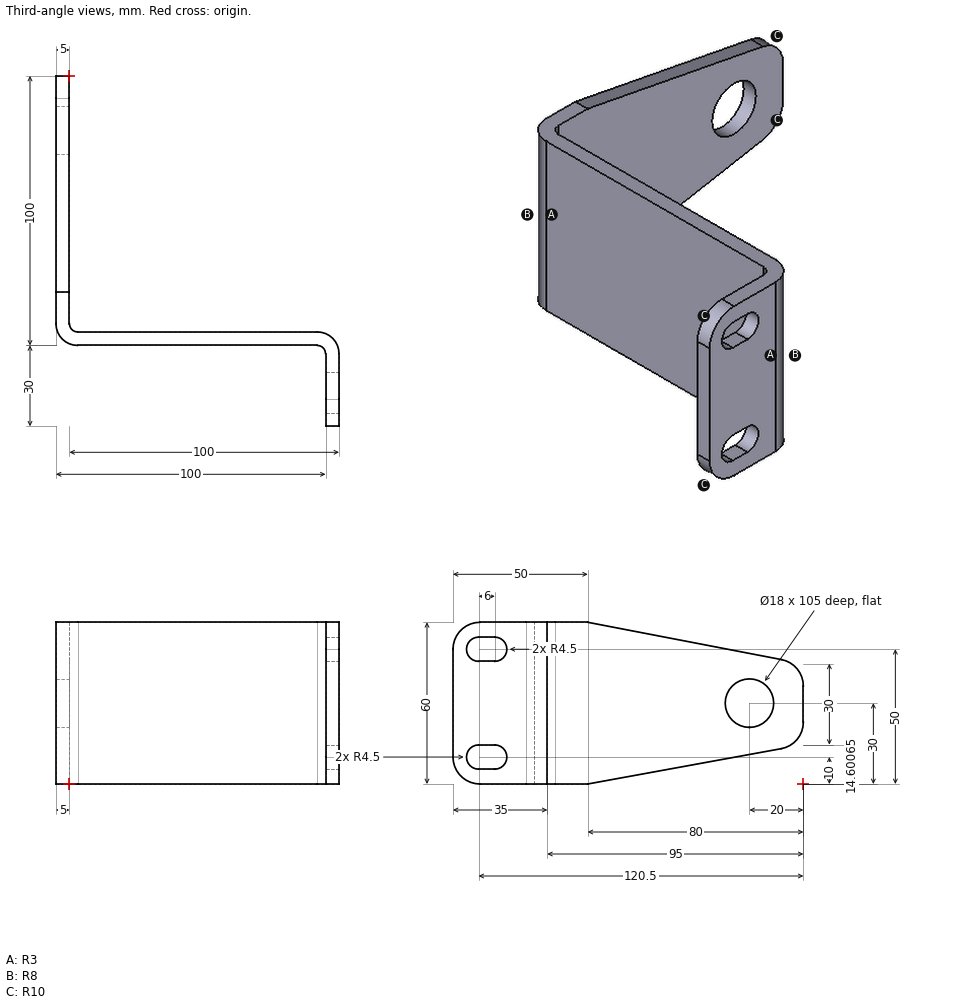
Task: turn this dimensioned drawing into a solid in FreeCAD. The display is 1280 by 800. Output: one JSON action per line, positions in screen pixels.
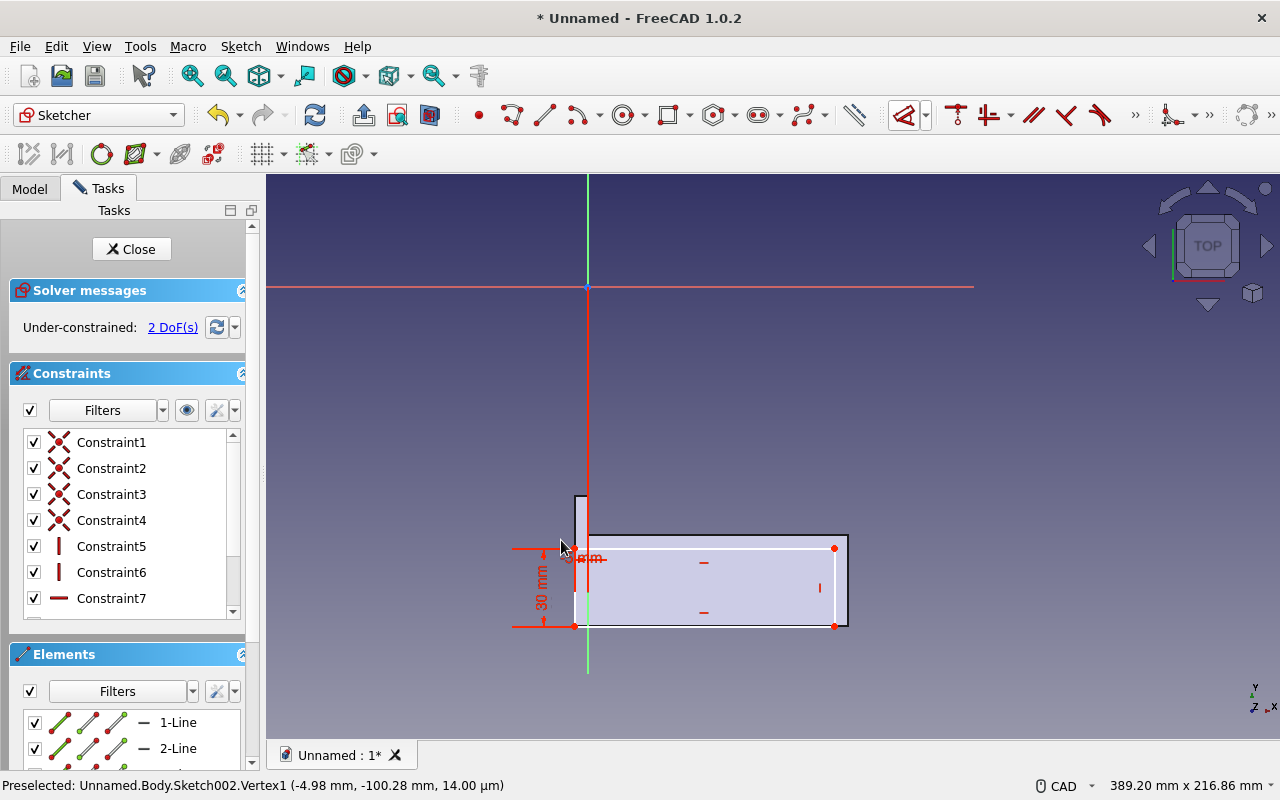
{"action": "left_click", "coordinate": [653, 627]}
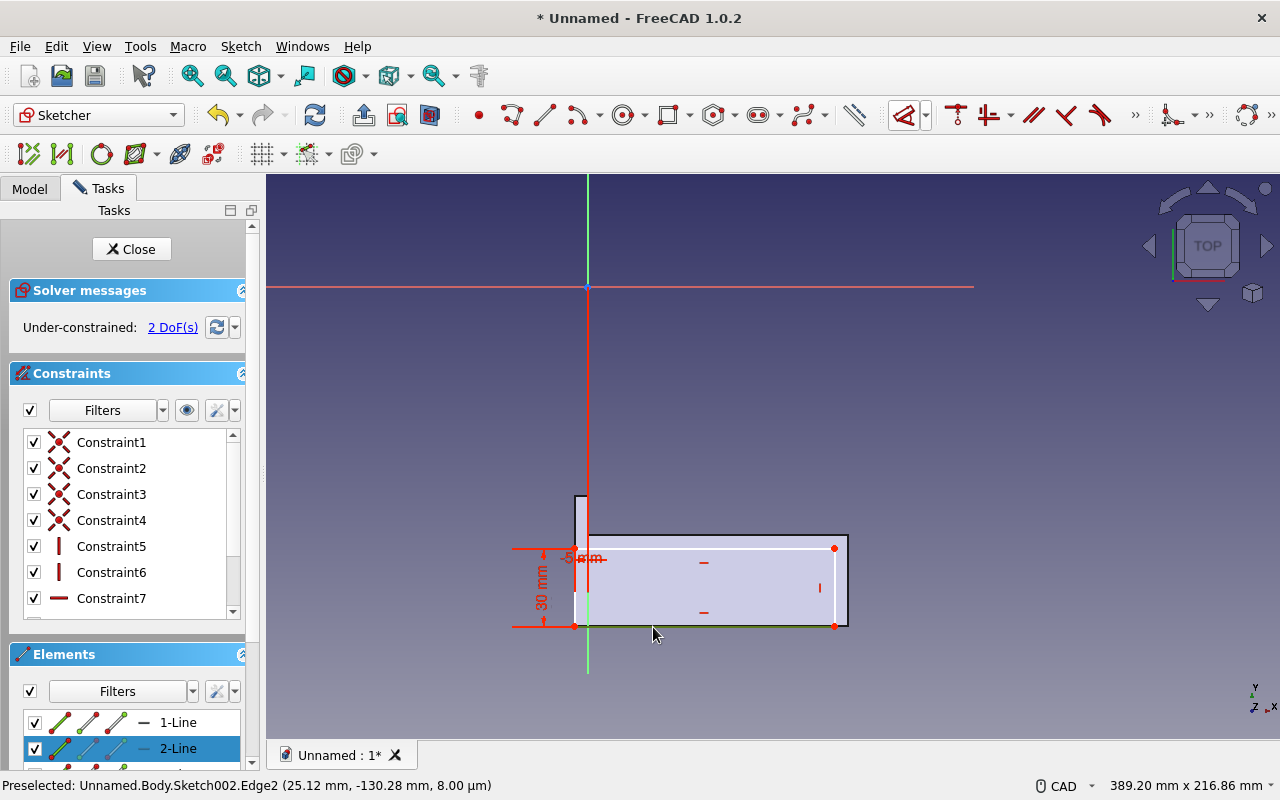
{"action": "key", "text": "l"}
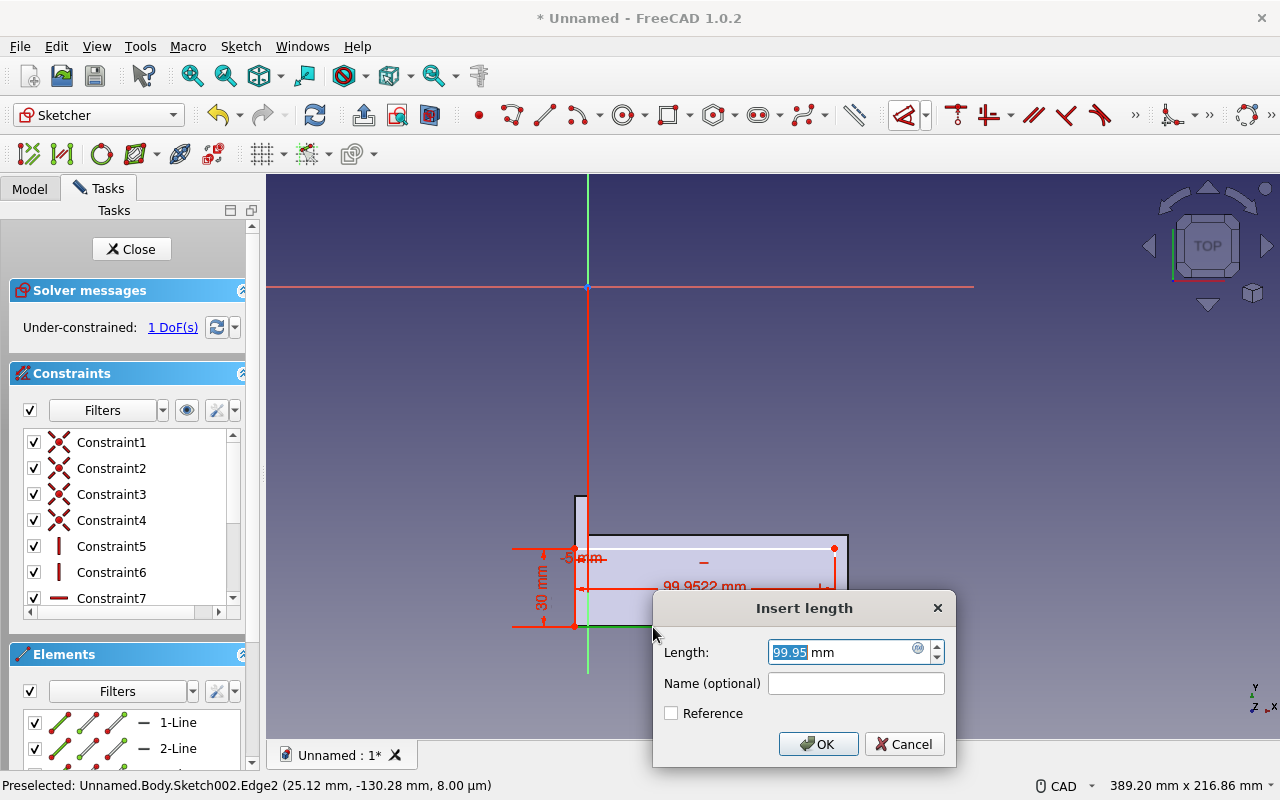
{"action": "type", "text": "100"}
{"action": "key", "text": "Return"}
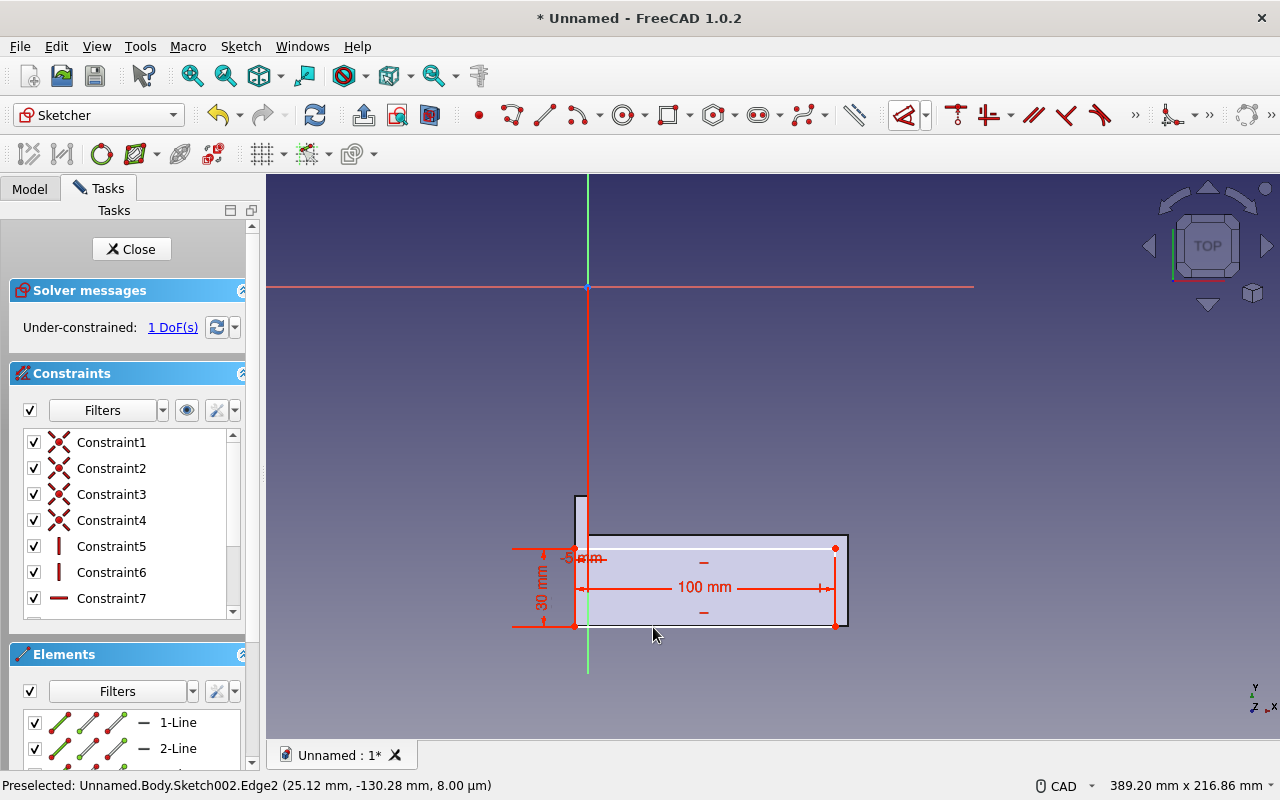
{"action": "left_click", "coordinate": [575, 549]}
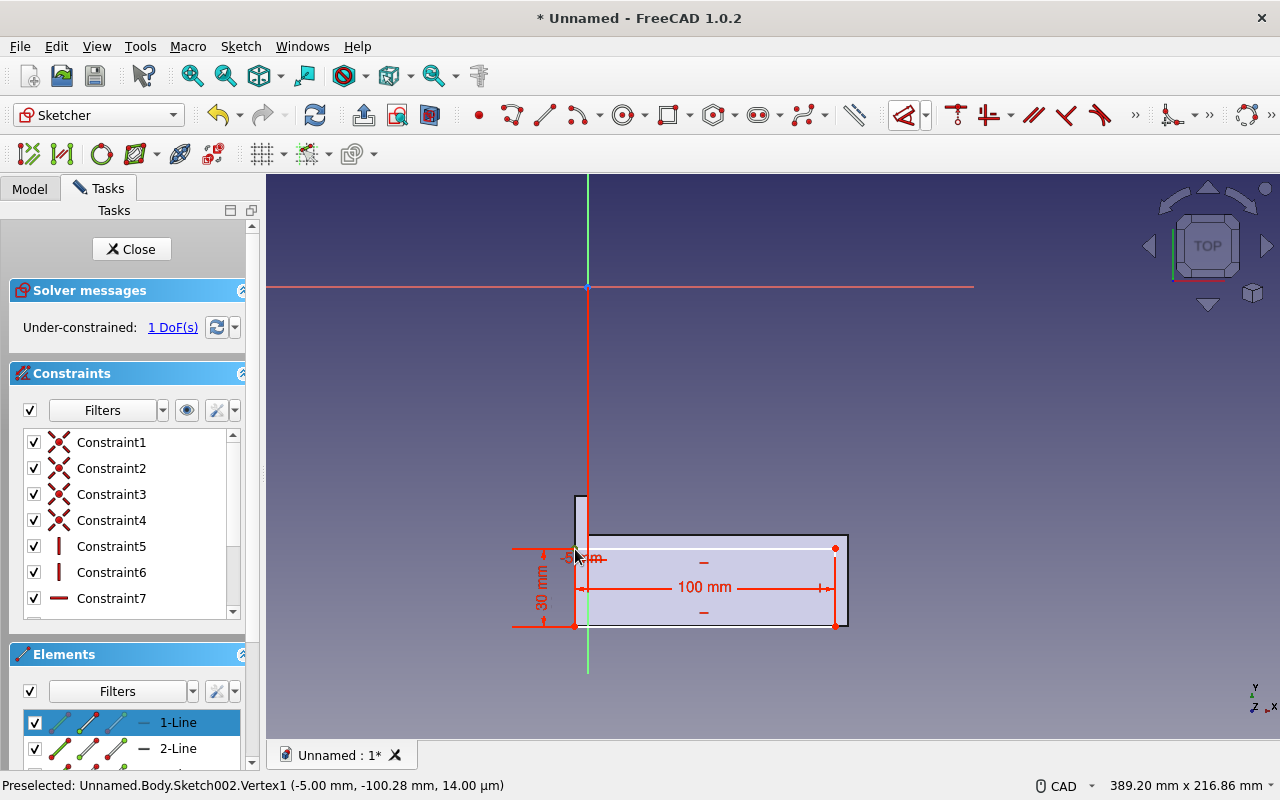
{"action": "left_click", "coordinate": [926, 116]}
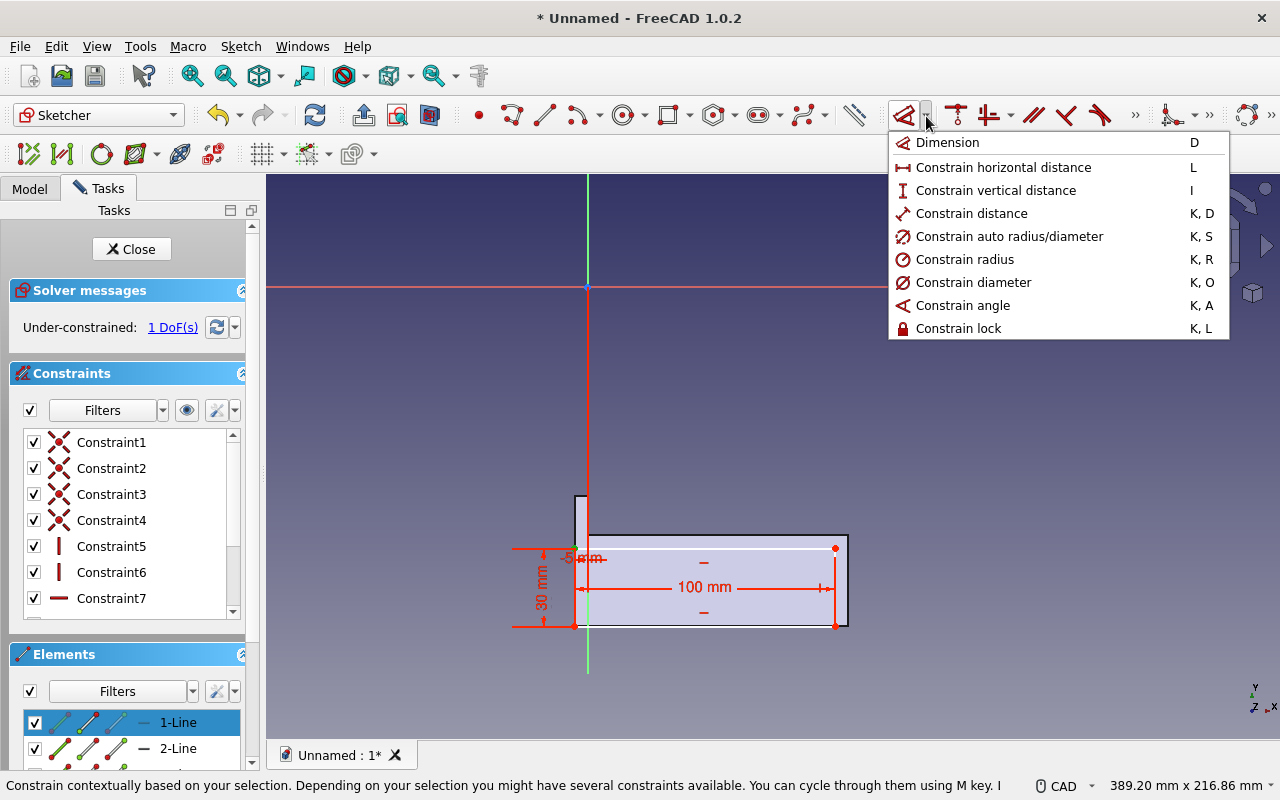
{"action": "left_click", "coordinate": [1059, 190]}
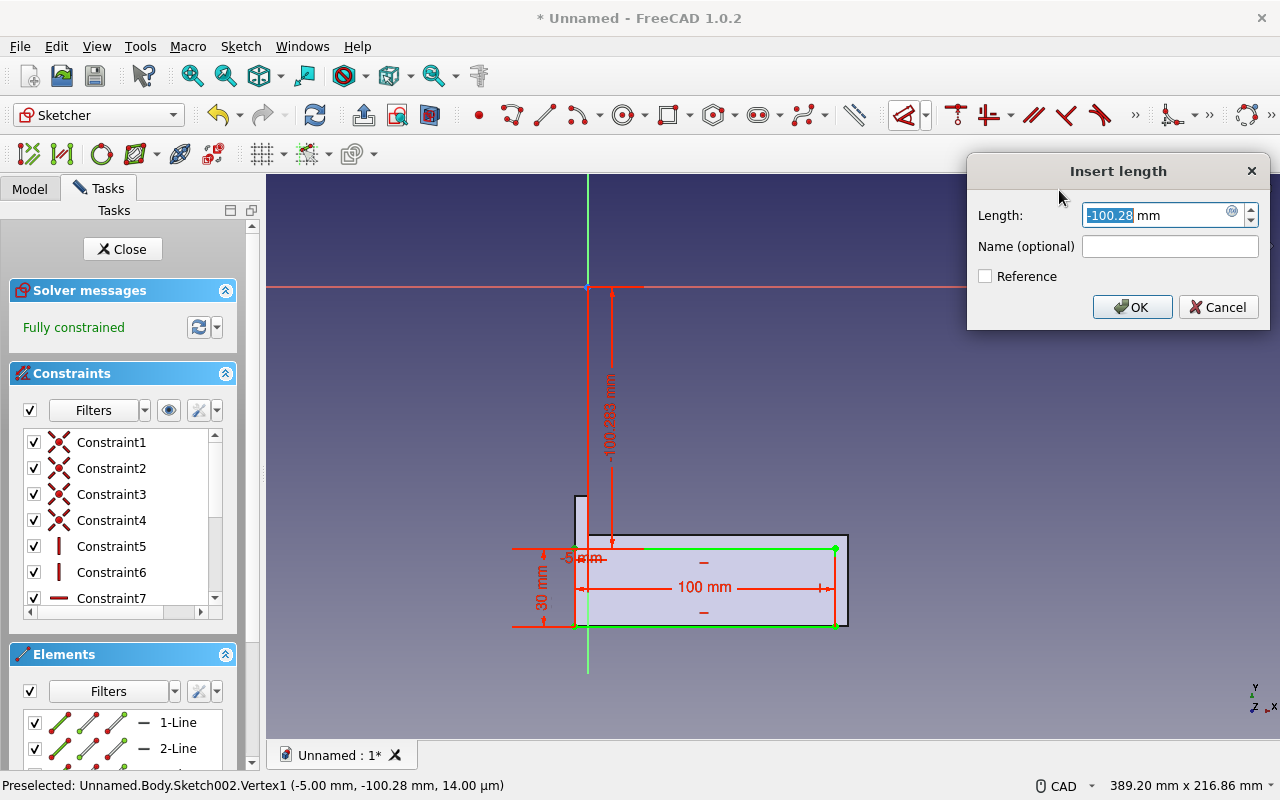
{"action": "type", "text": "-100"}
{"action": "key", "text": "Return"}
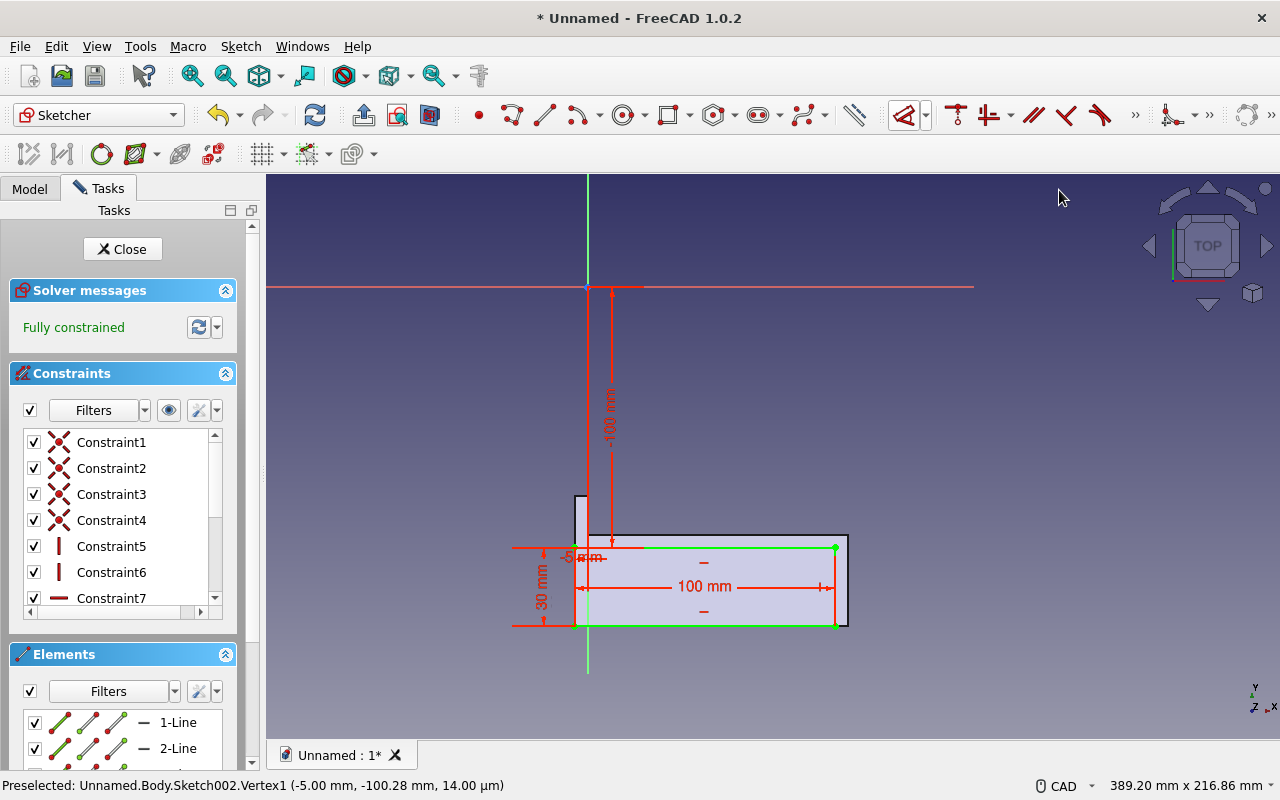
{"action": "left_click", "coordinate": [123, 249]}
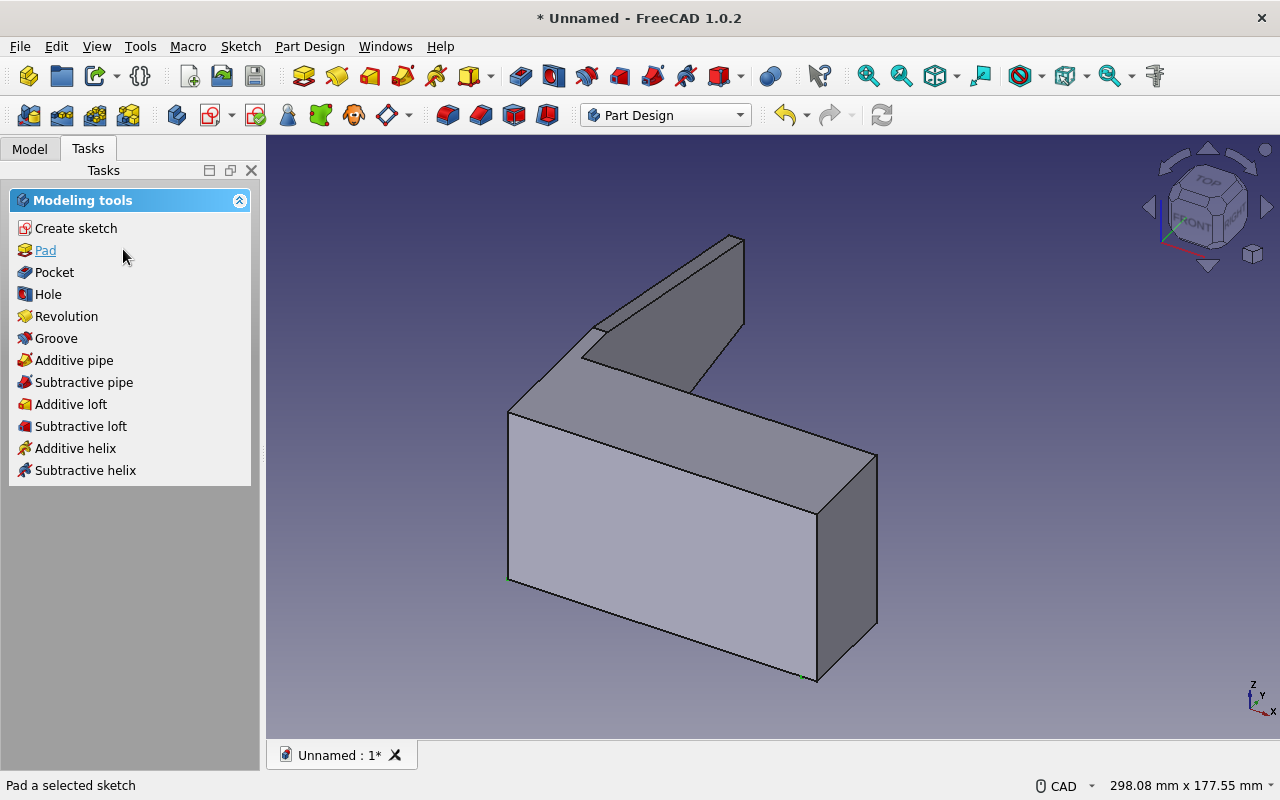
{"action": "left_click", "coordinate": [521, 76]}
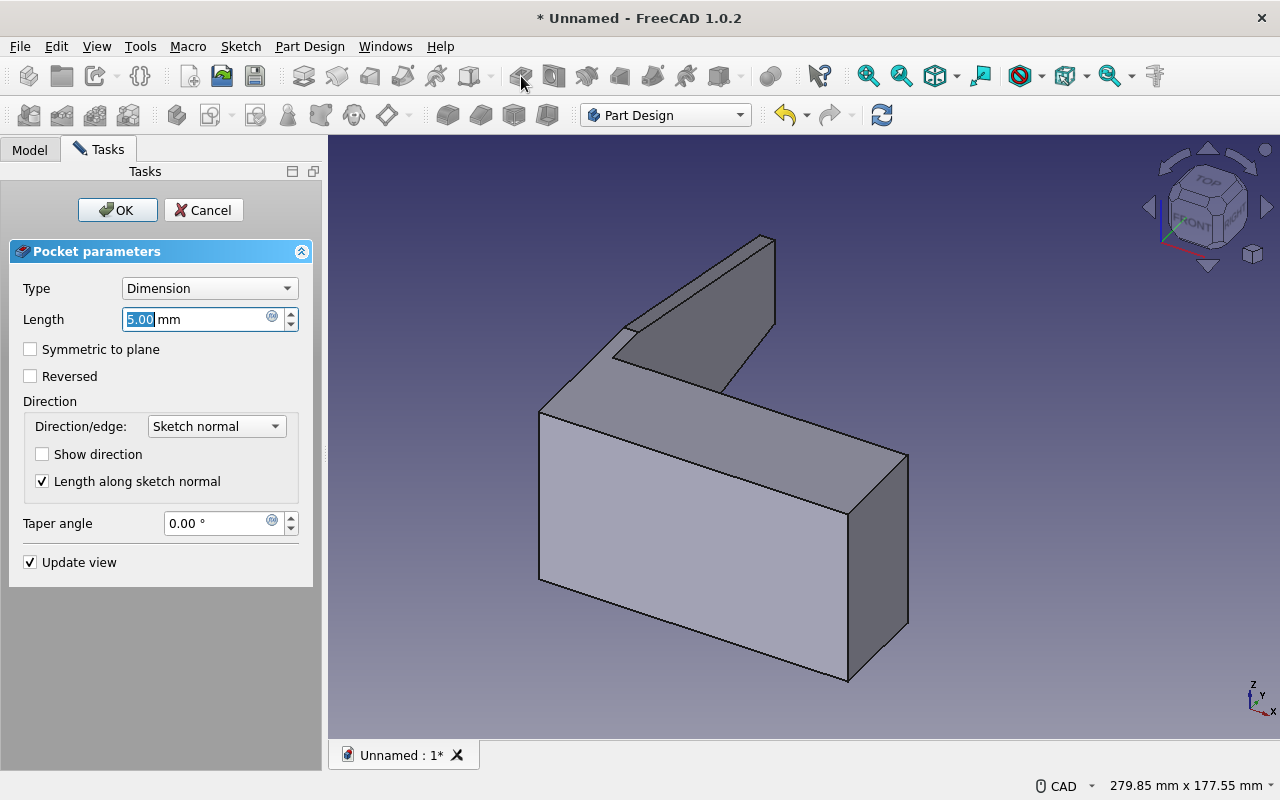
{"action": "left_click", "coordinate": [210, 288]}